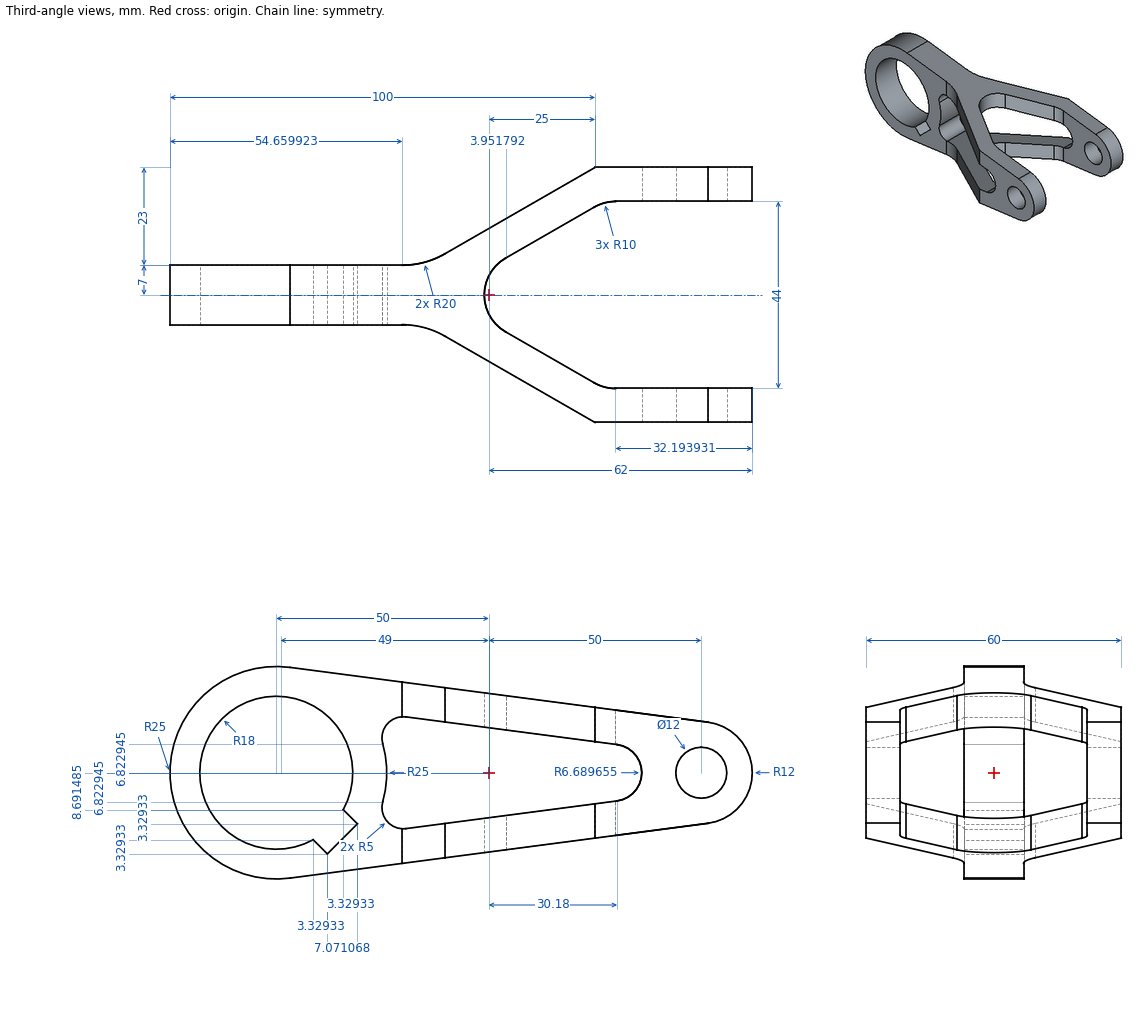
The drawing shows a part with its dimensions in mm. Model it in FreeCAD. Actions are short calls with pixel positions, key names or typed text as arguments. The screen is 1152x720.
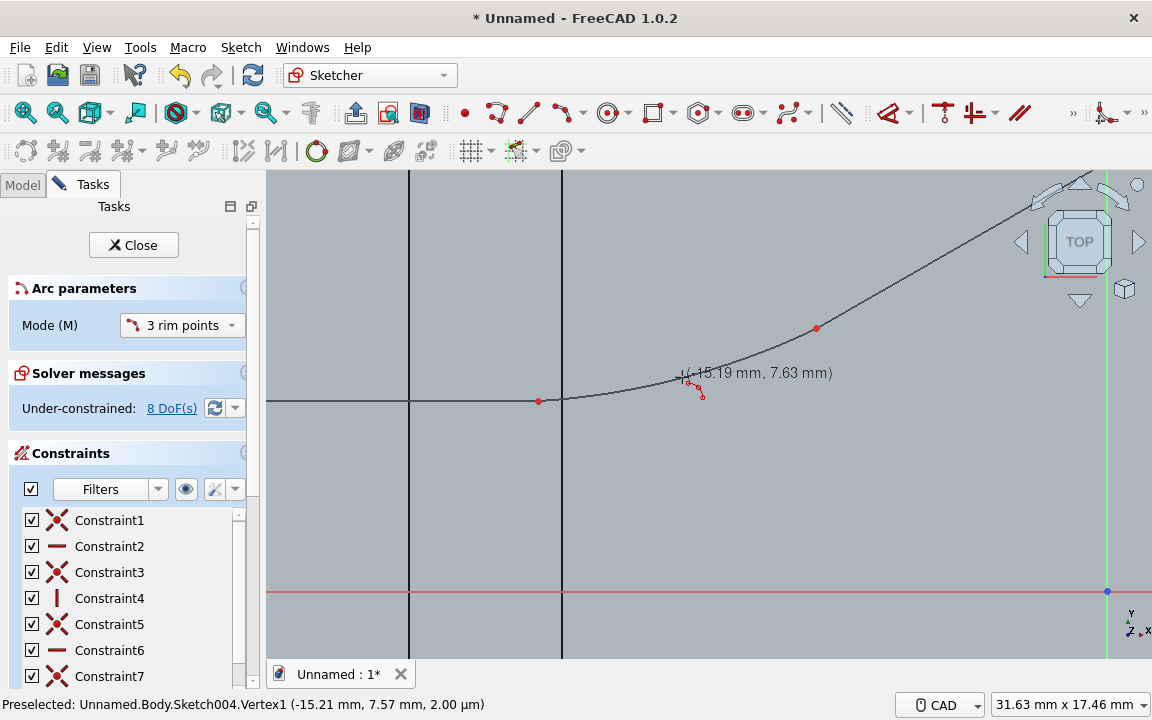
click(498, 114)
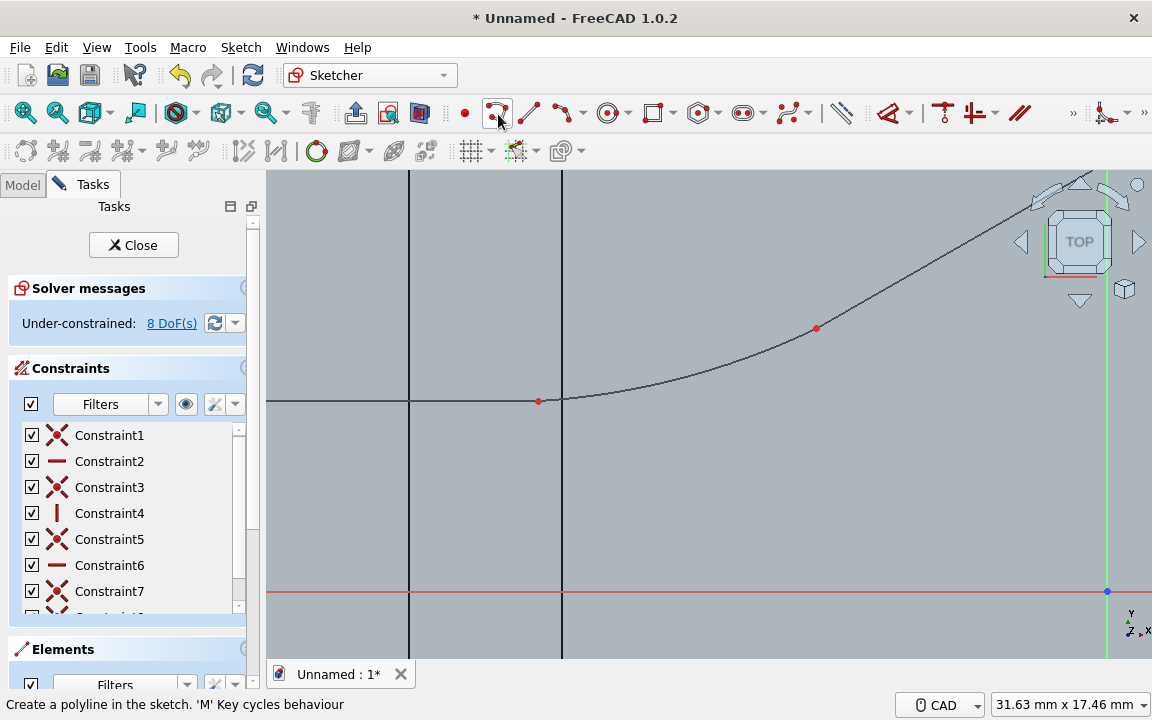
scroll(687, 379, down, 9)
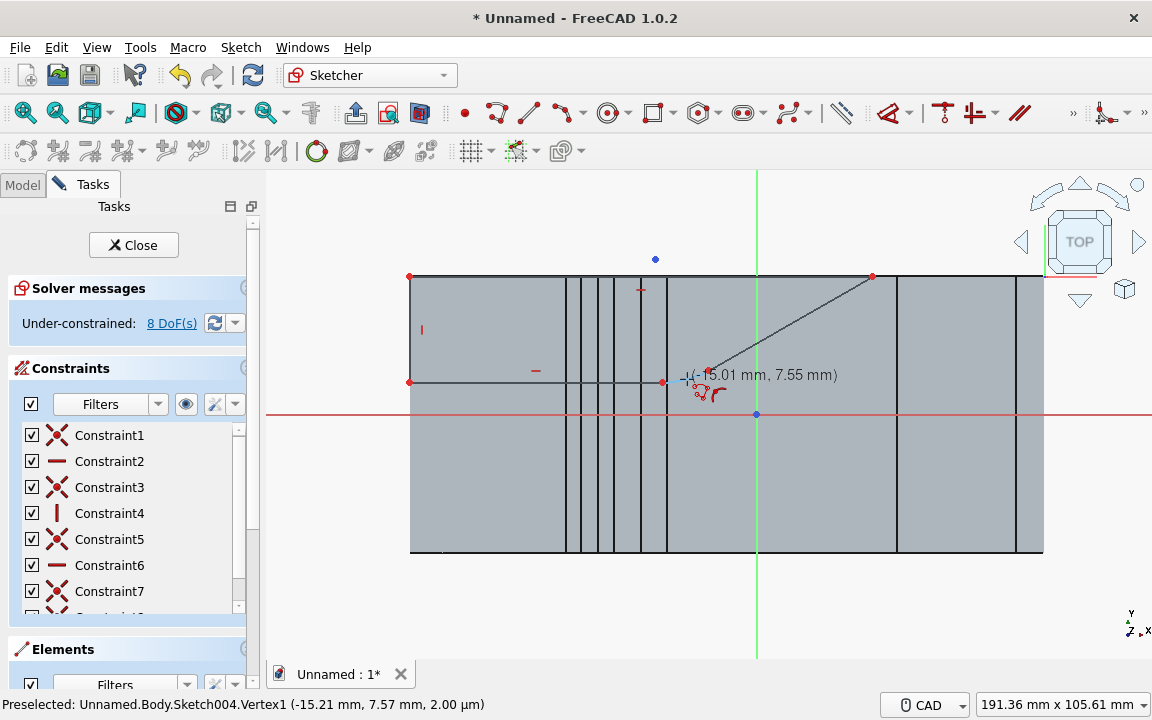
click(663, 447)
click(410, 447)
click(410, 553)
click(873, 553)
click(709, 459)
right_click(709, 459)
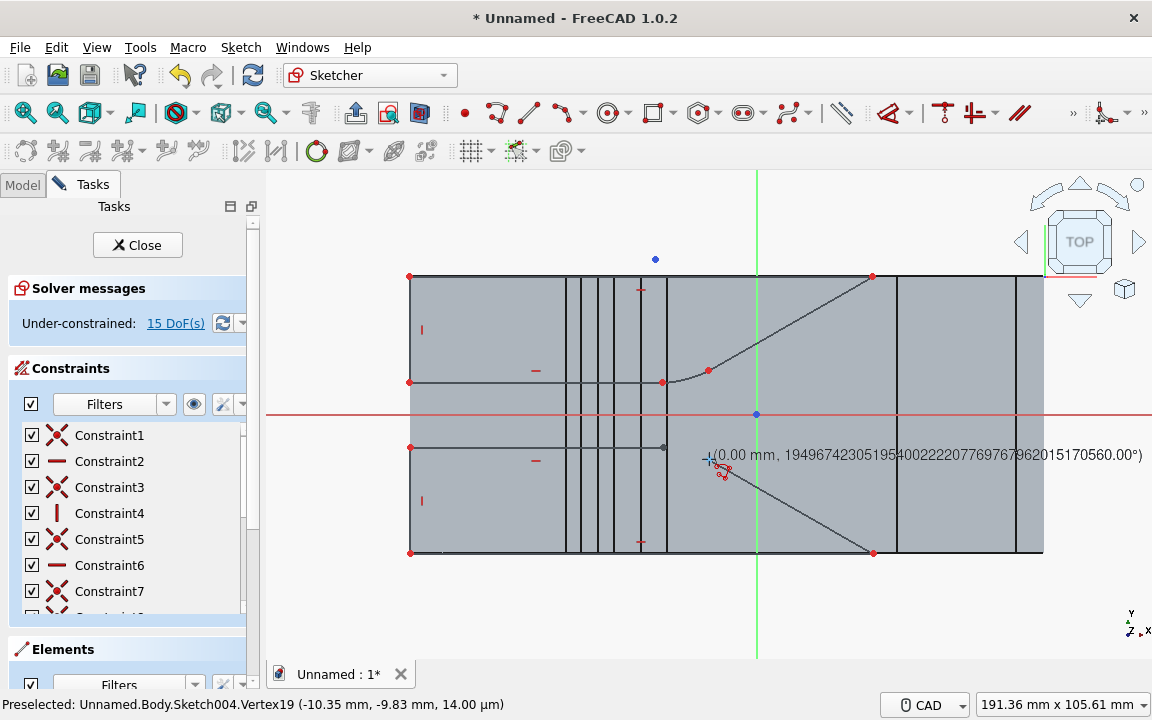
click(562, 114)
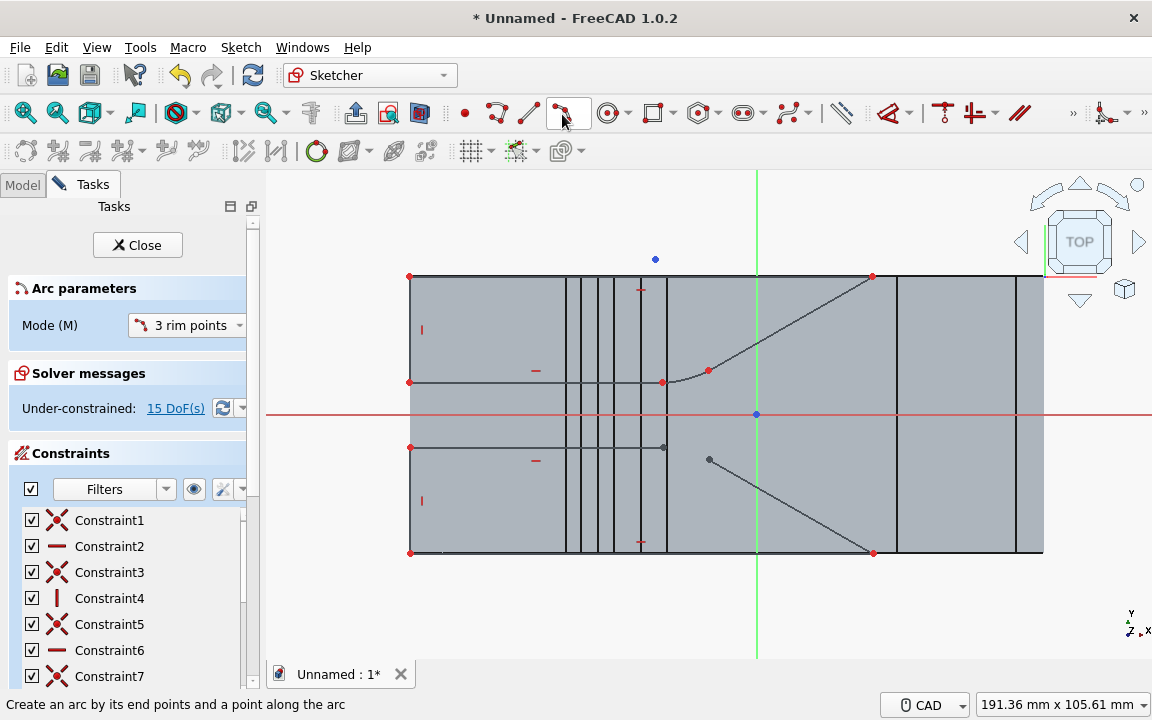
click(709, 460)
click(663, 448)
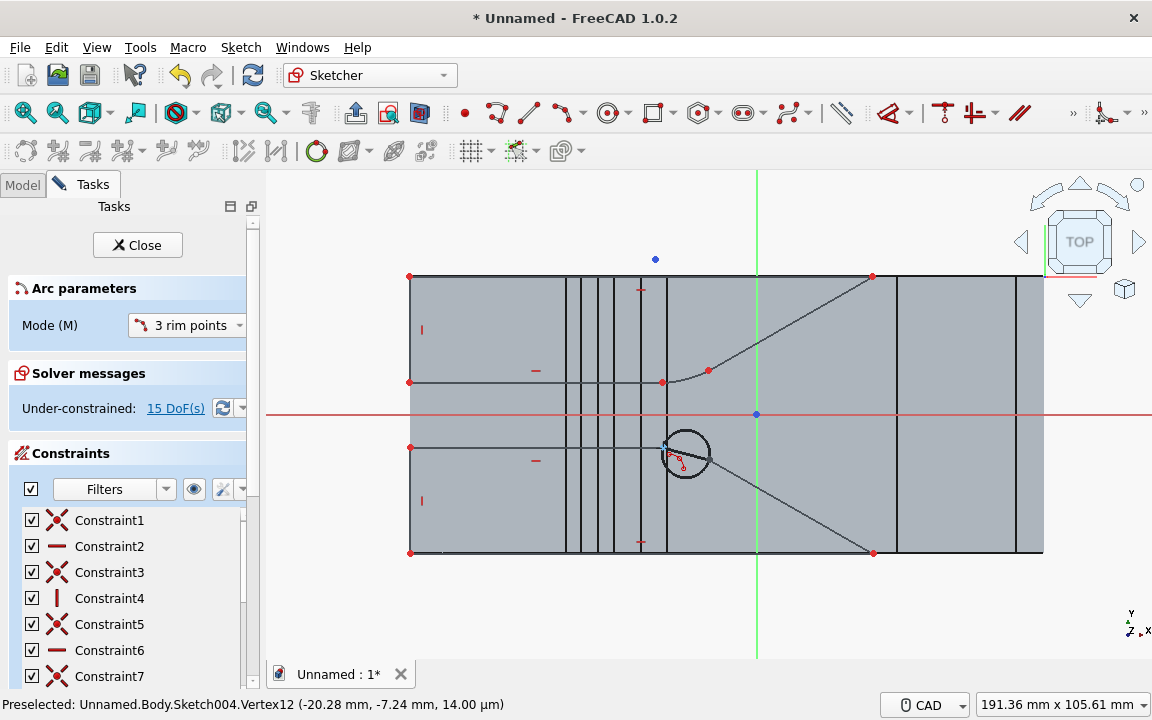
scroll(687, 450, up, 9)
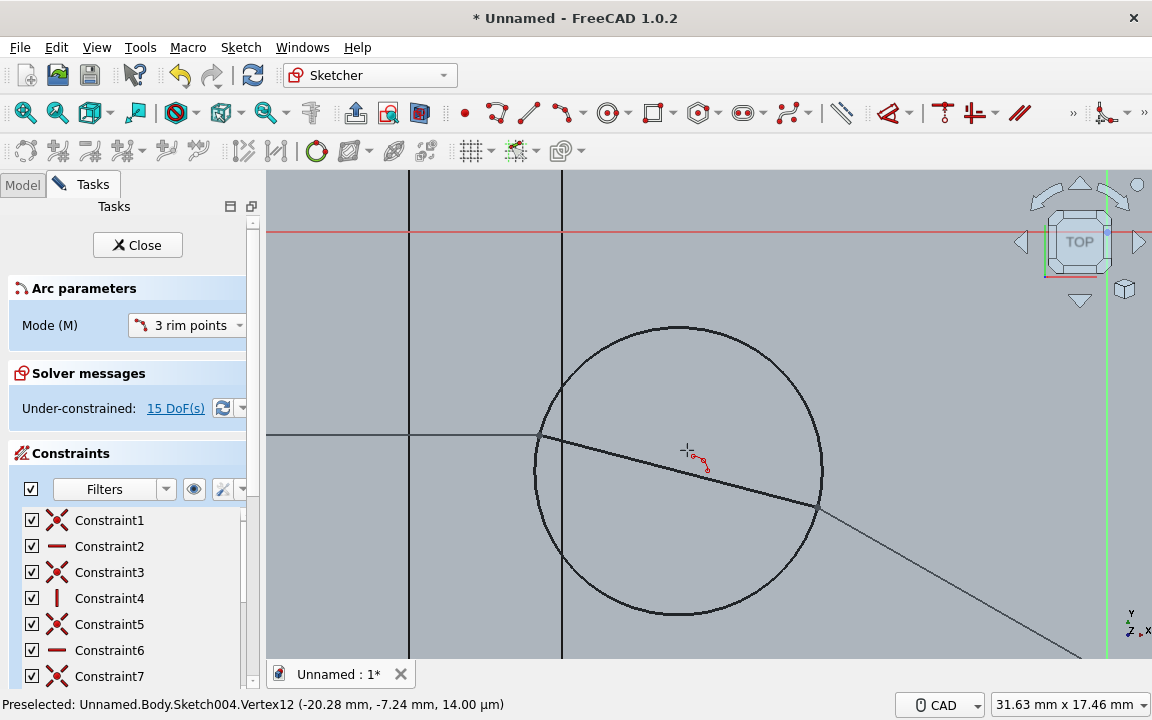
click(682, 447)
key(Escape)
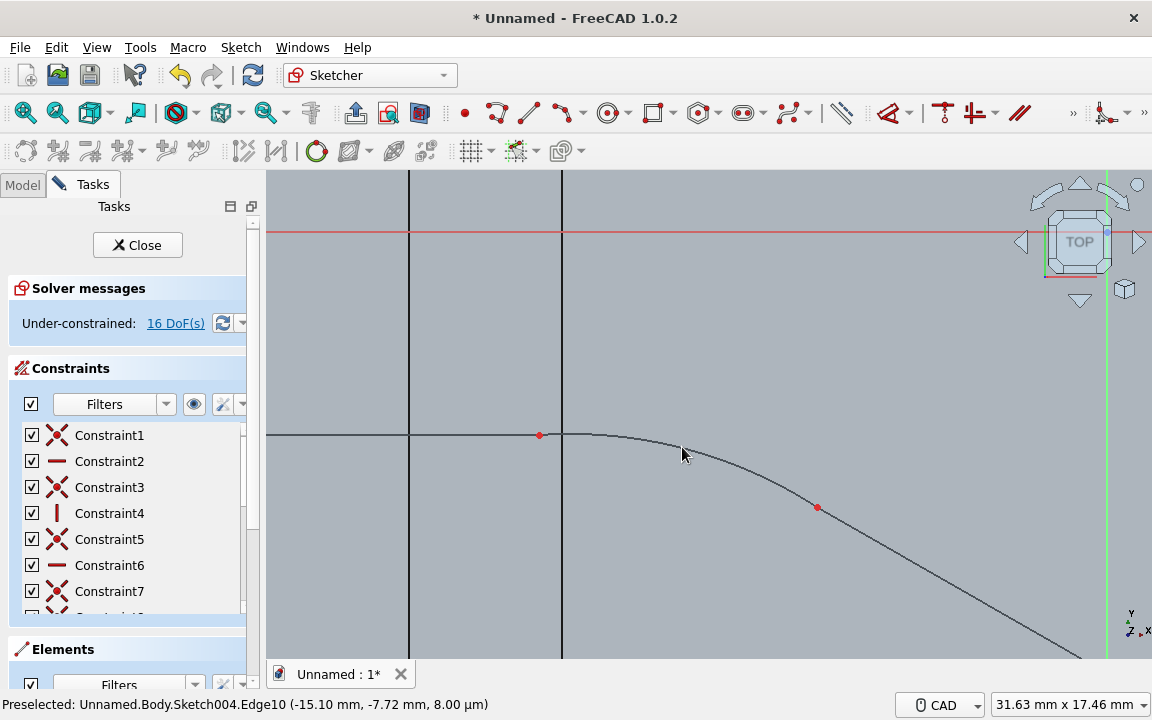
scroll(687, 451, down, 9)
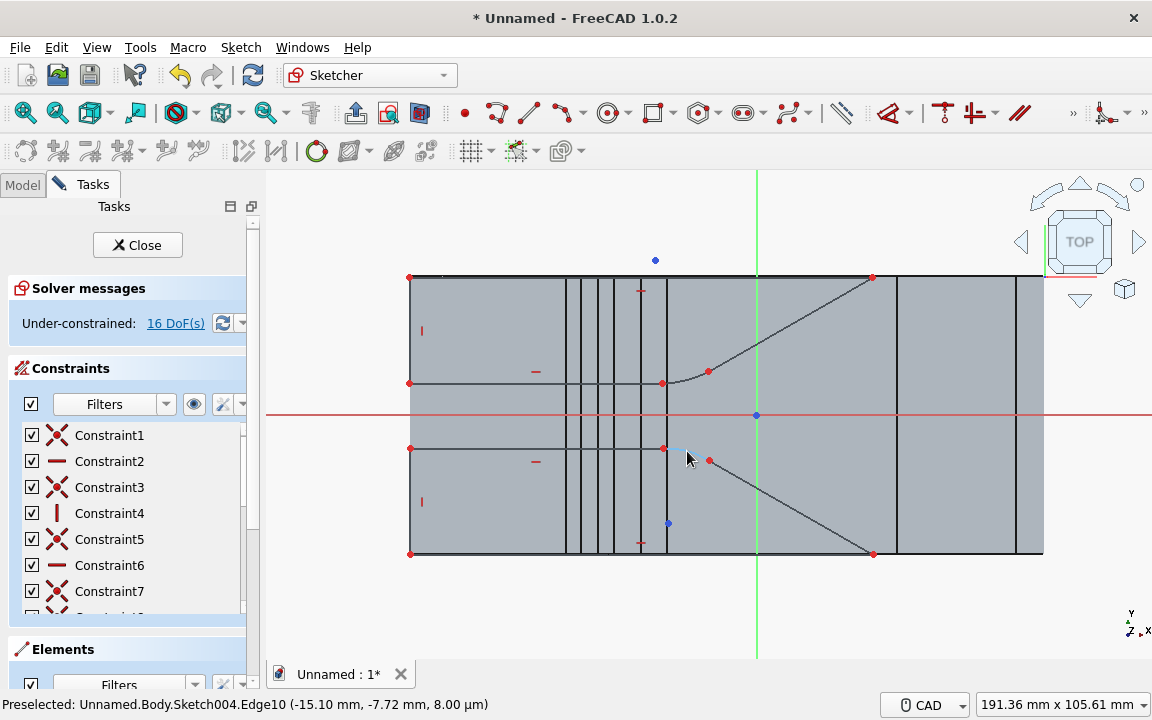
click(824, 306)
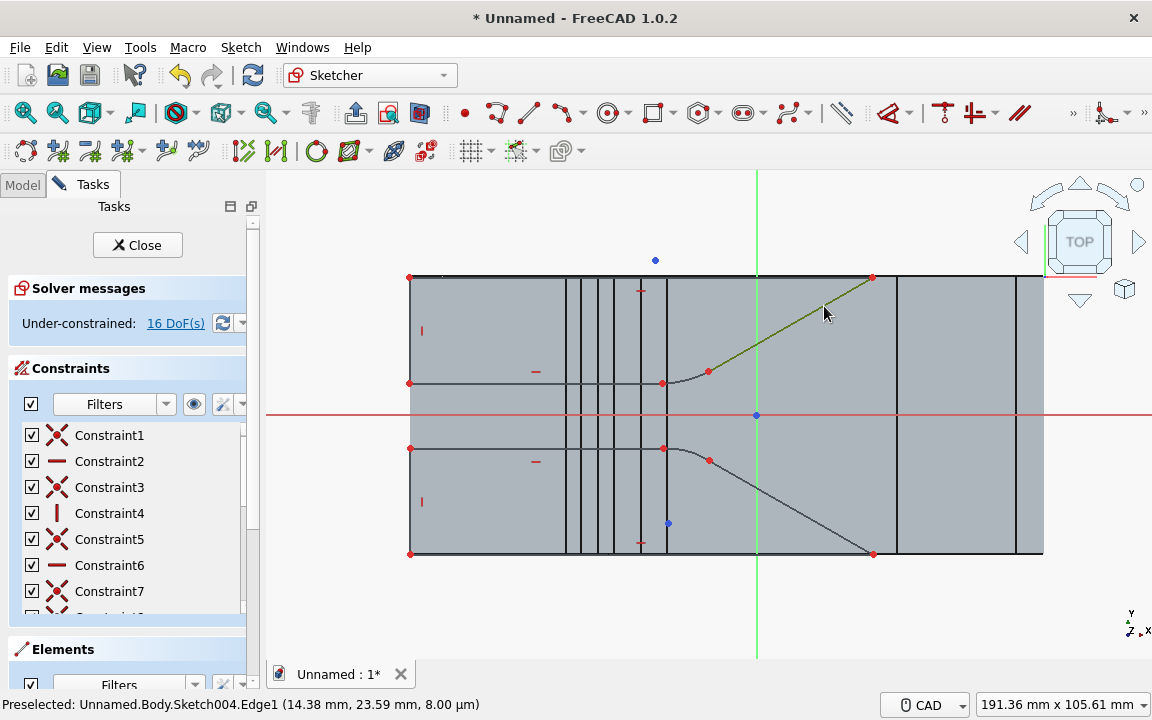
click(677, 382)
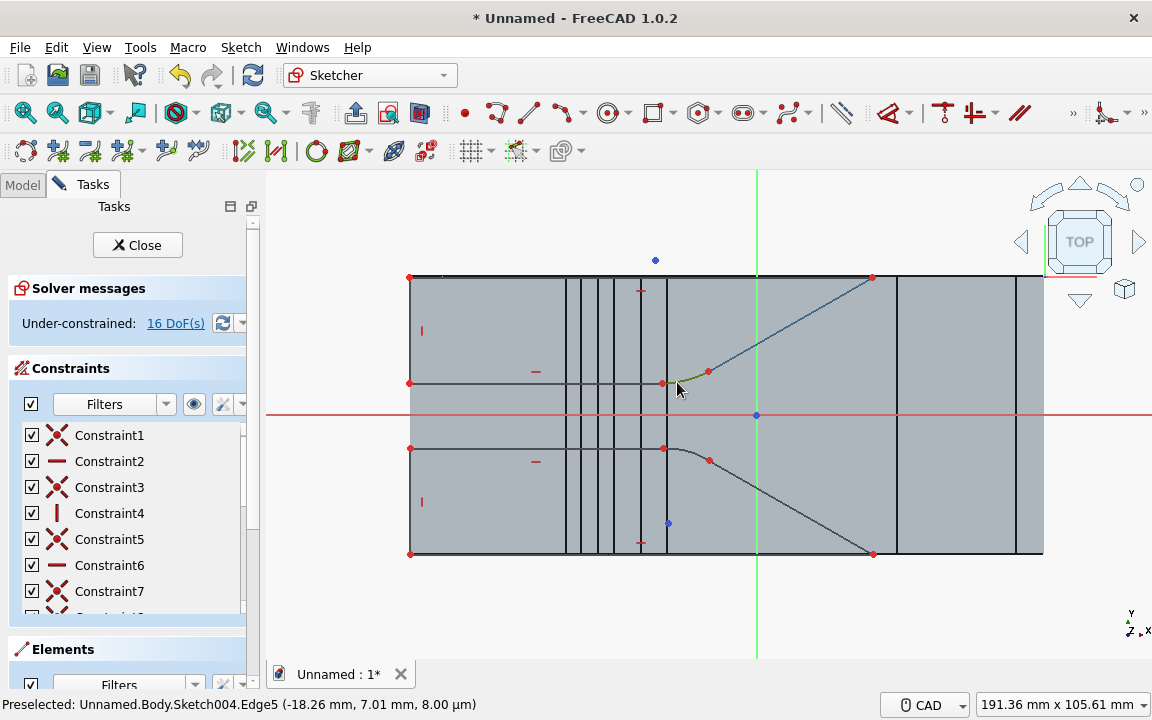
key(t)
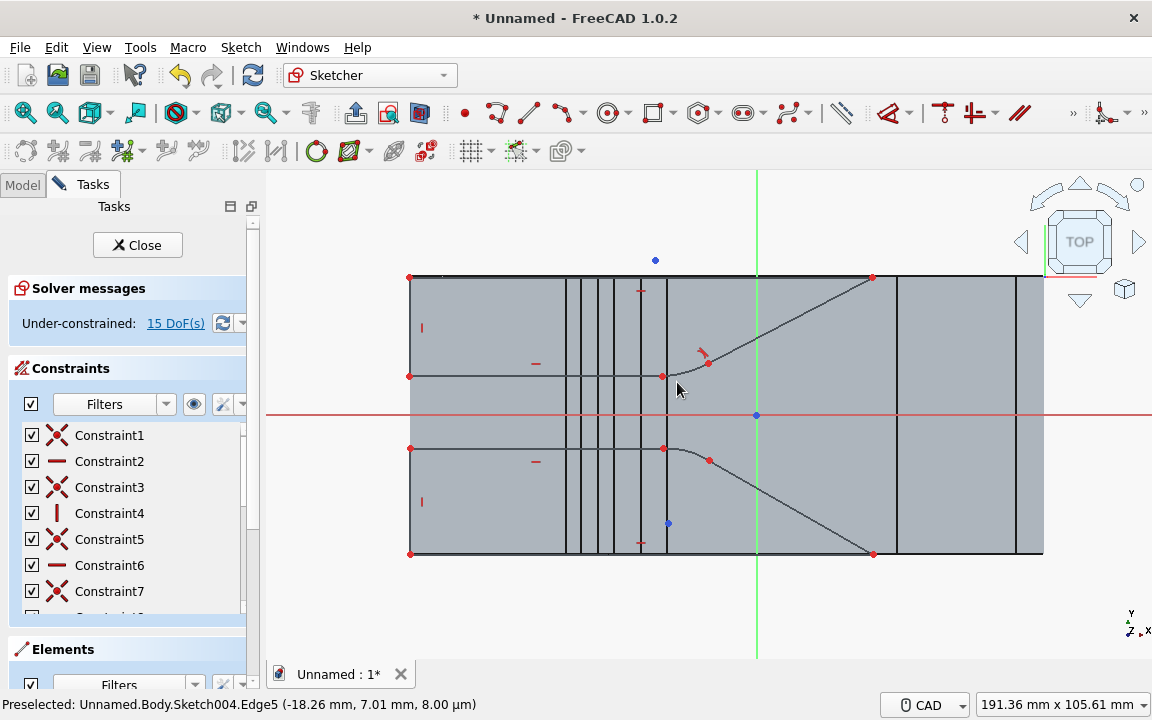
click(486, 376)